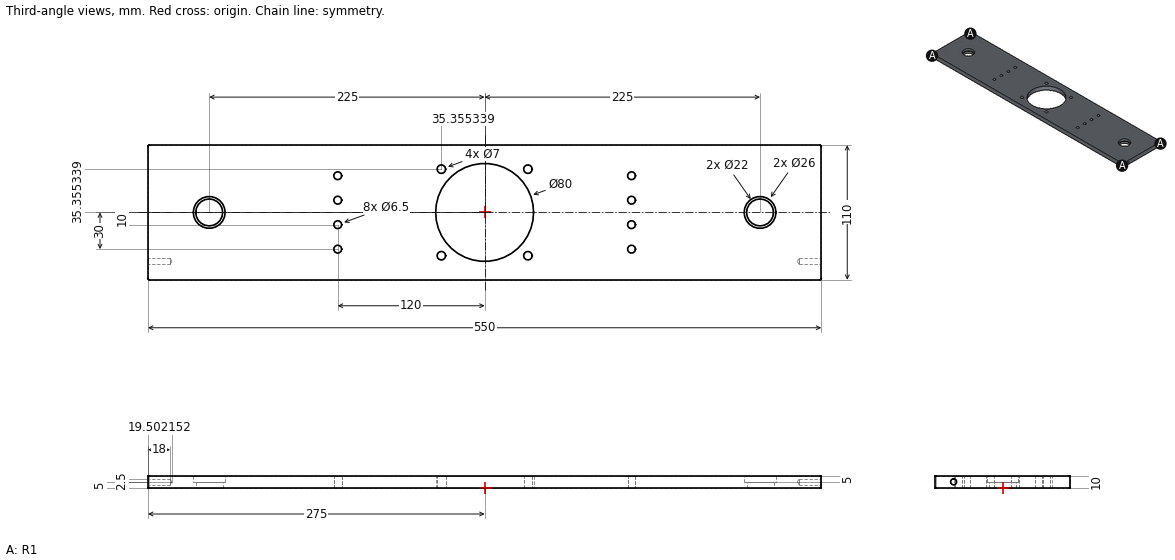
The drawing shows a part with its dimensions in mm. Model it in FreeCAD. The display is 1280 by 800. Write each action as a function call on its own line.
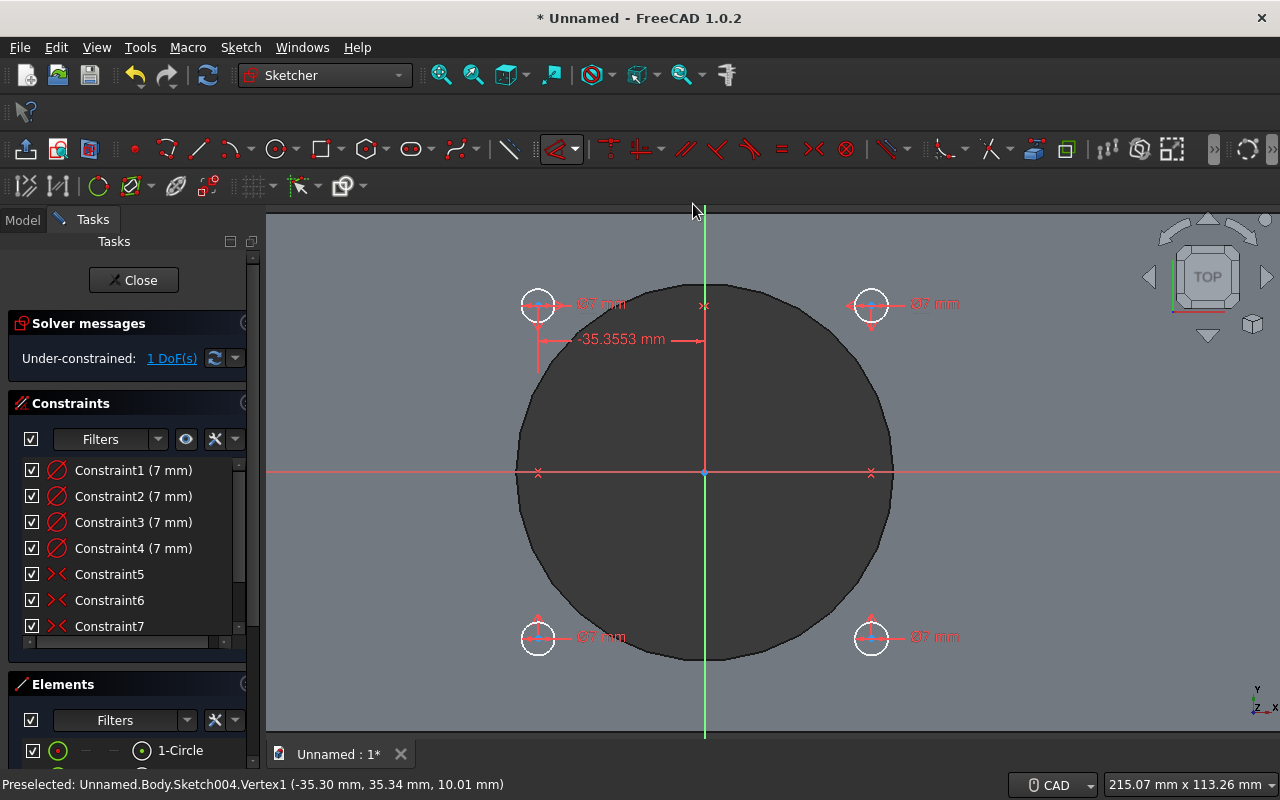
click(538, 306)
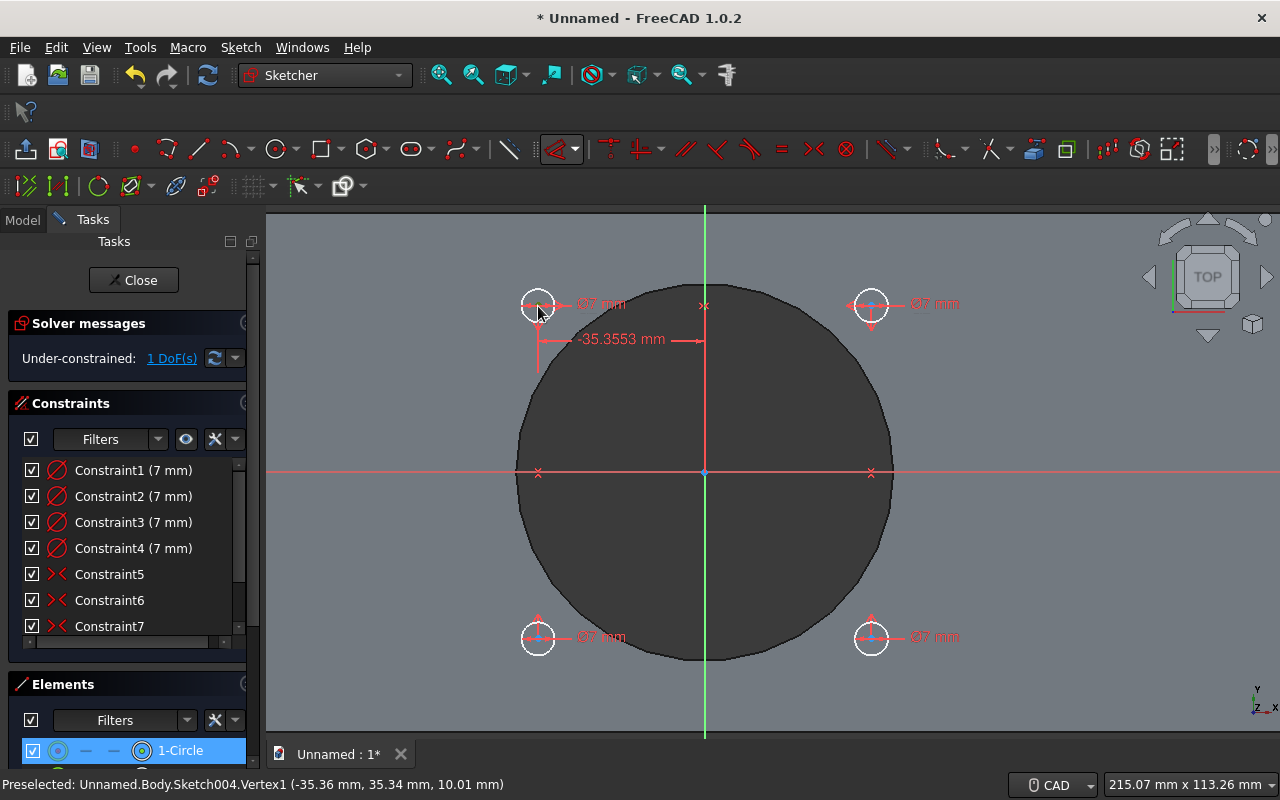
key(i)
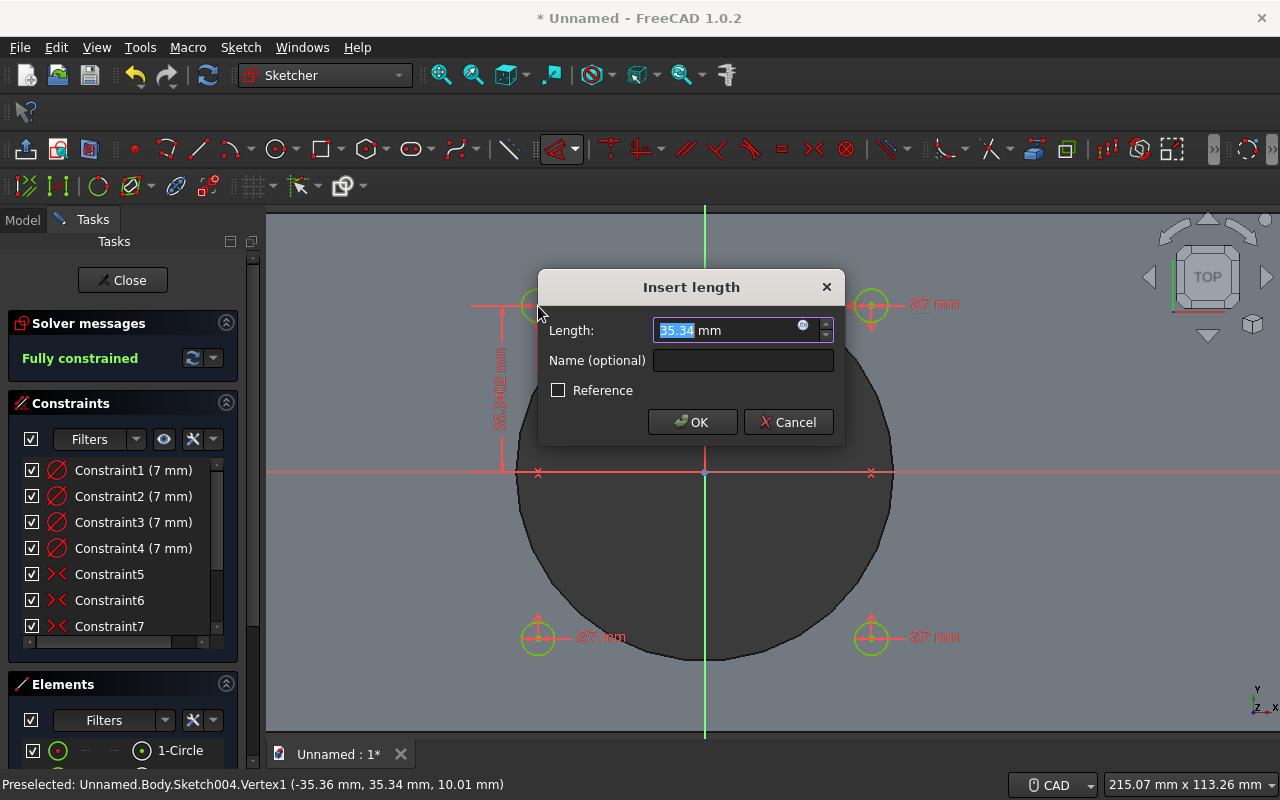
text(35.355339)
key(Return)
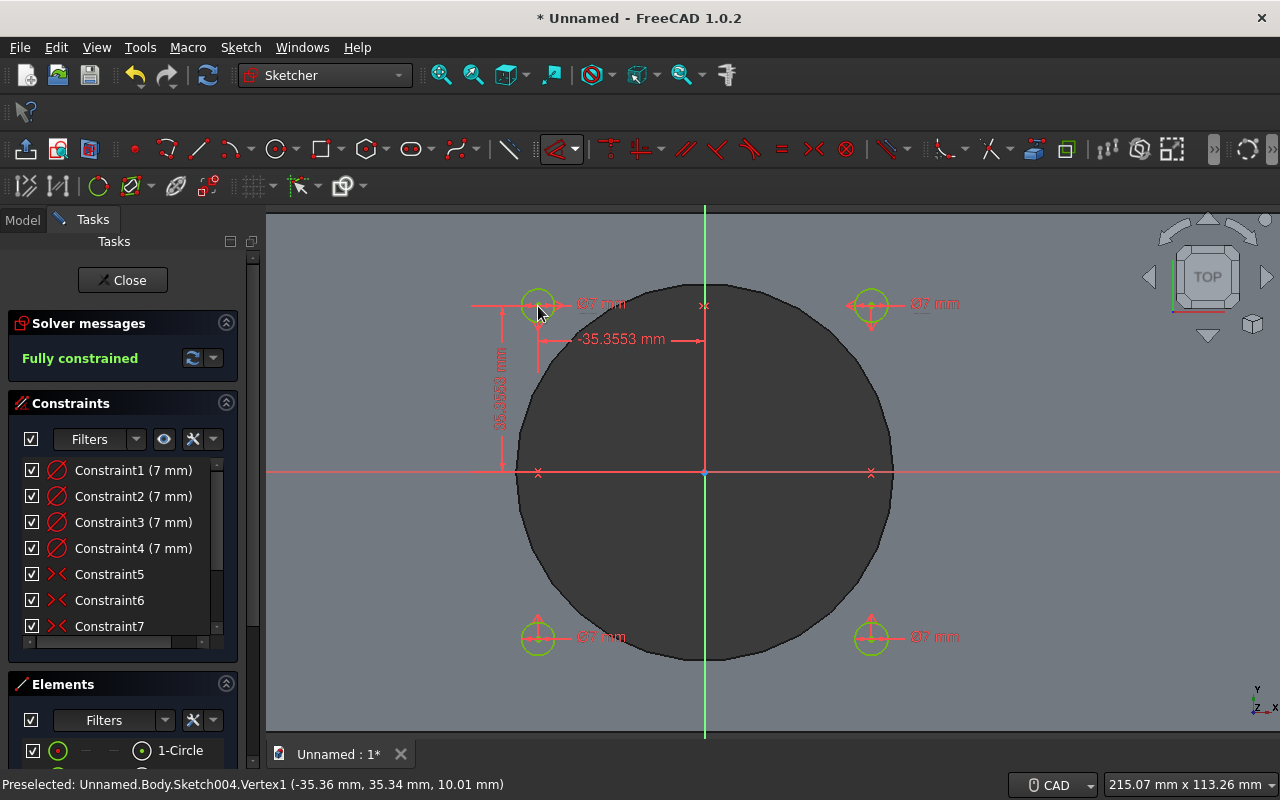
click(123, 280)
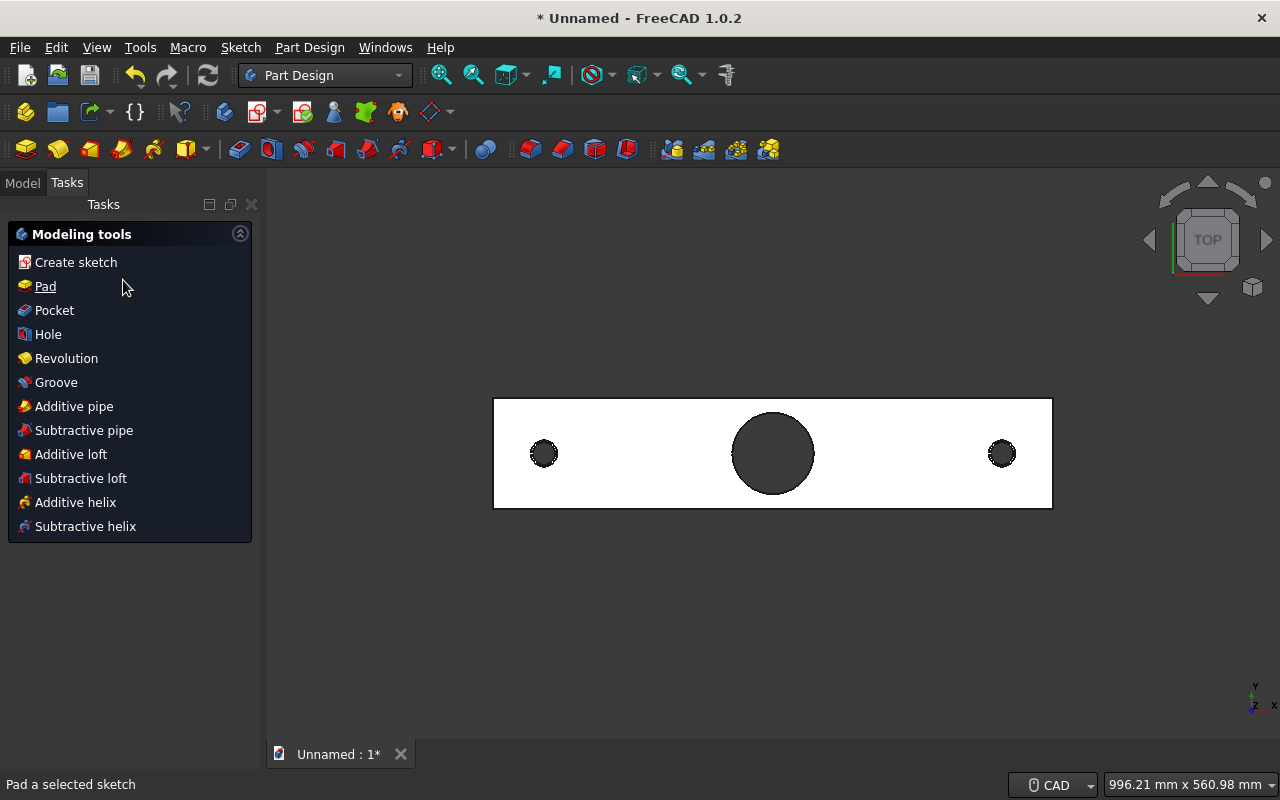
click(240, 150)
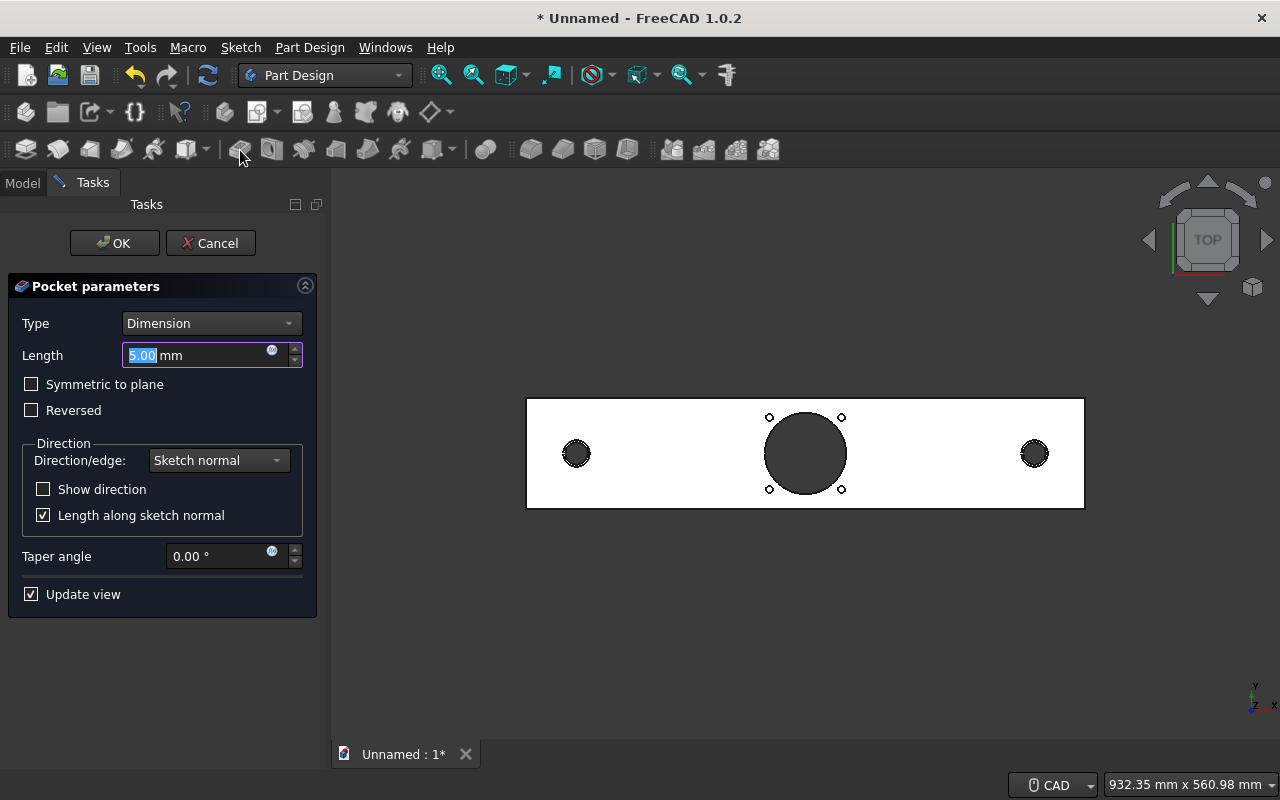
click(212, 324)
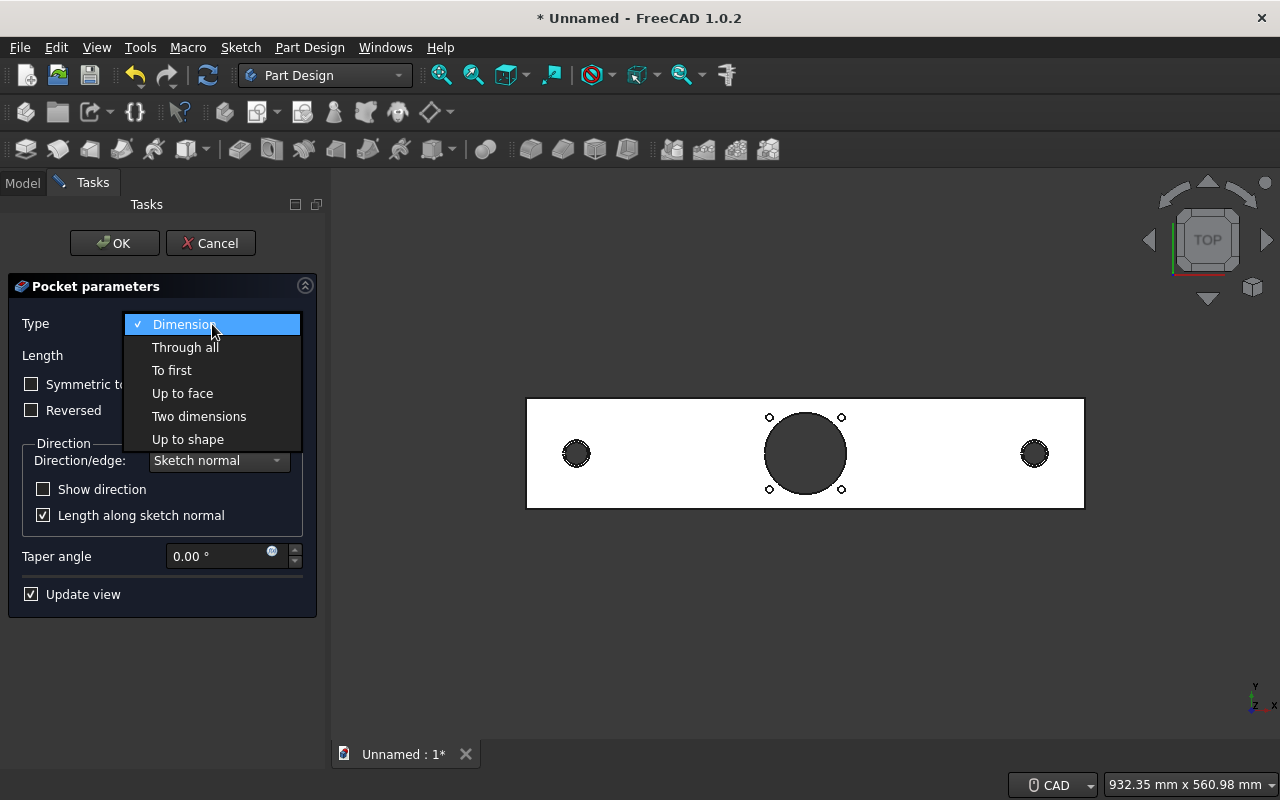
click(212, 348)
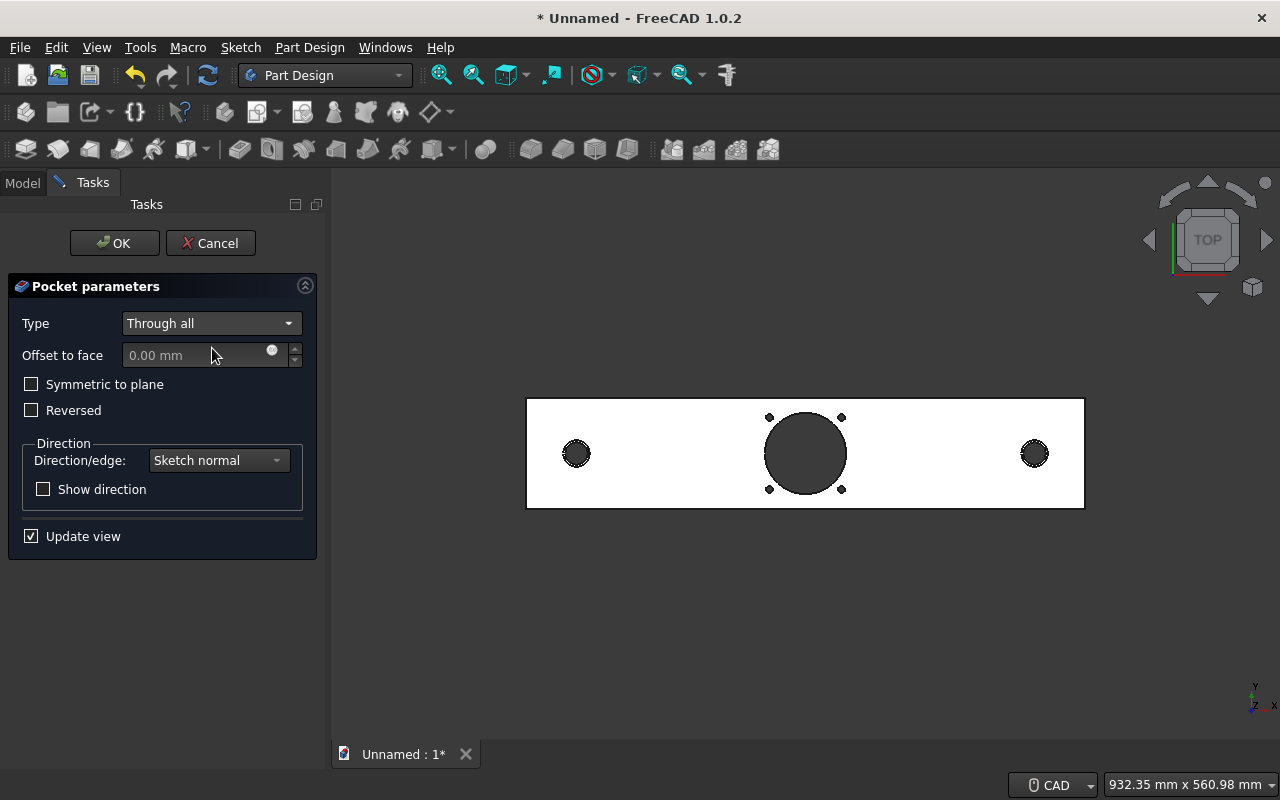
click(115, 243)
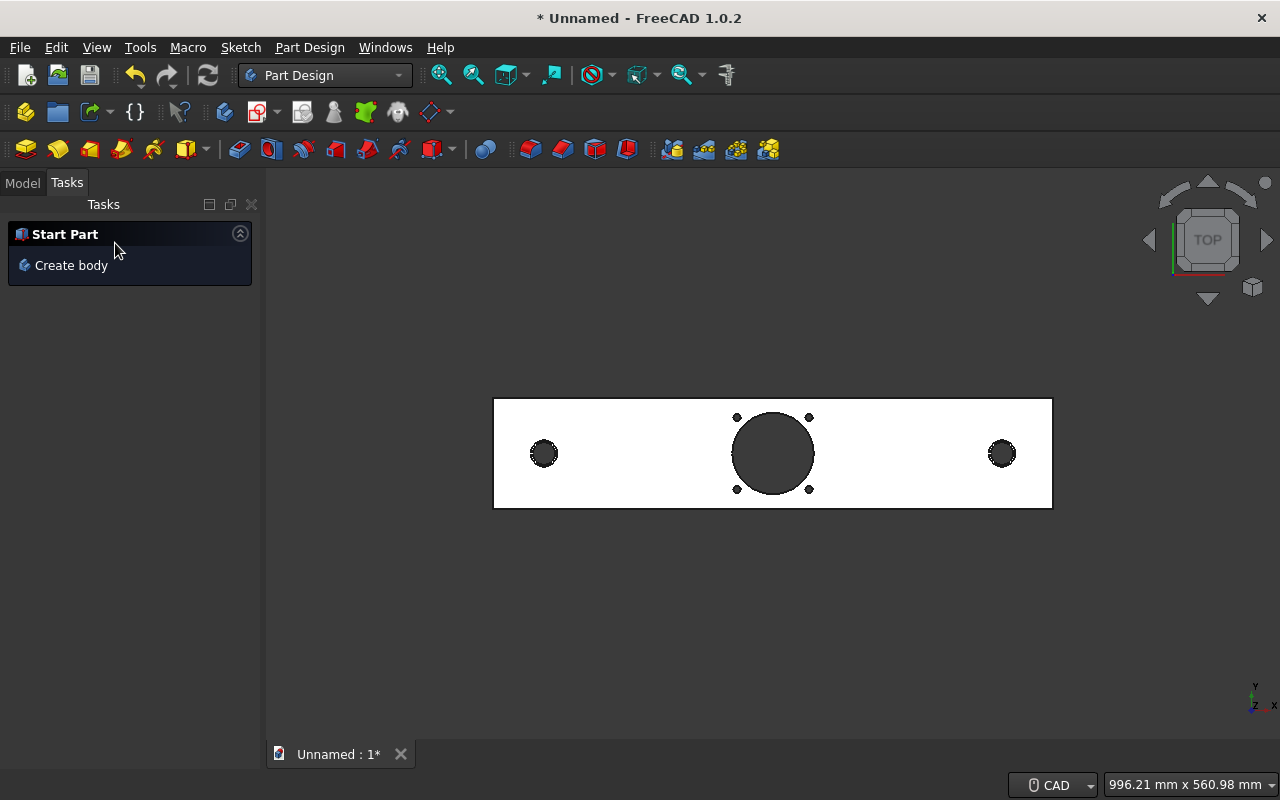
click(613, 452)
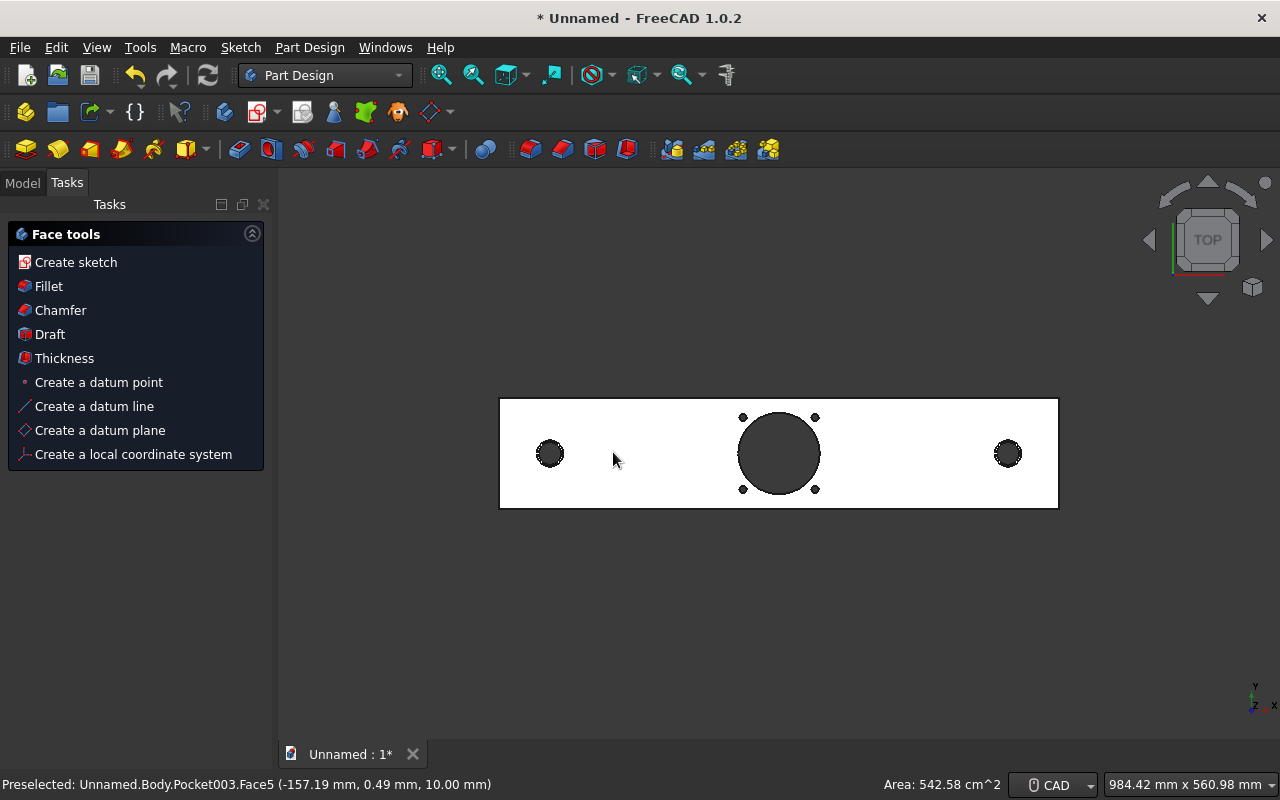
click(258, 112)